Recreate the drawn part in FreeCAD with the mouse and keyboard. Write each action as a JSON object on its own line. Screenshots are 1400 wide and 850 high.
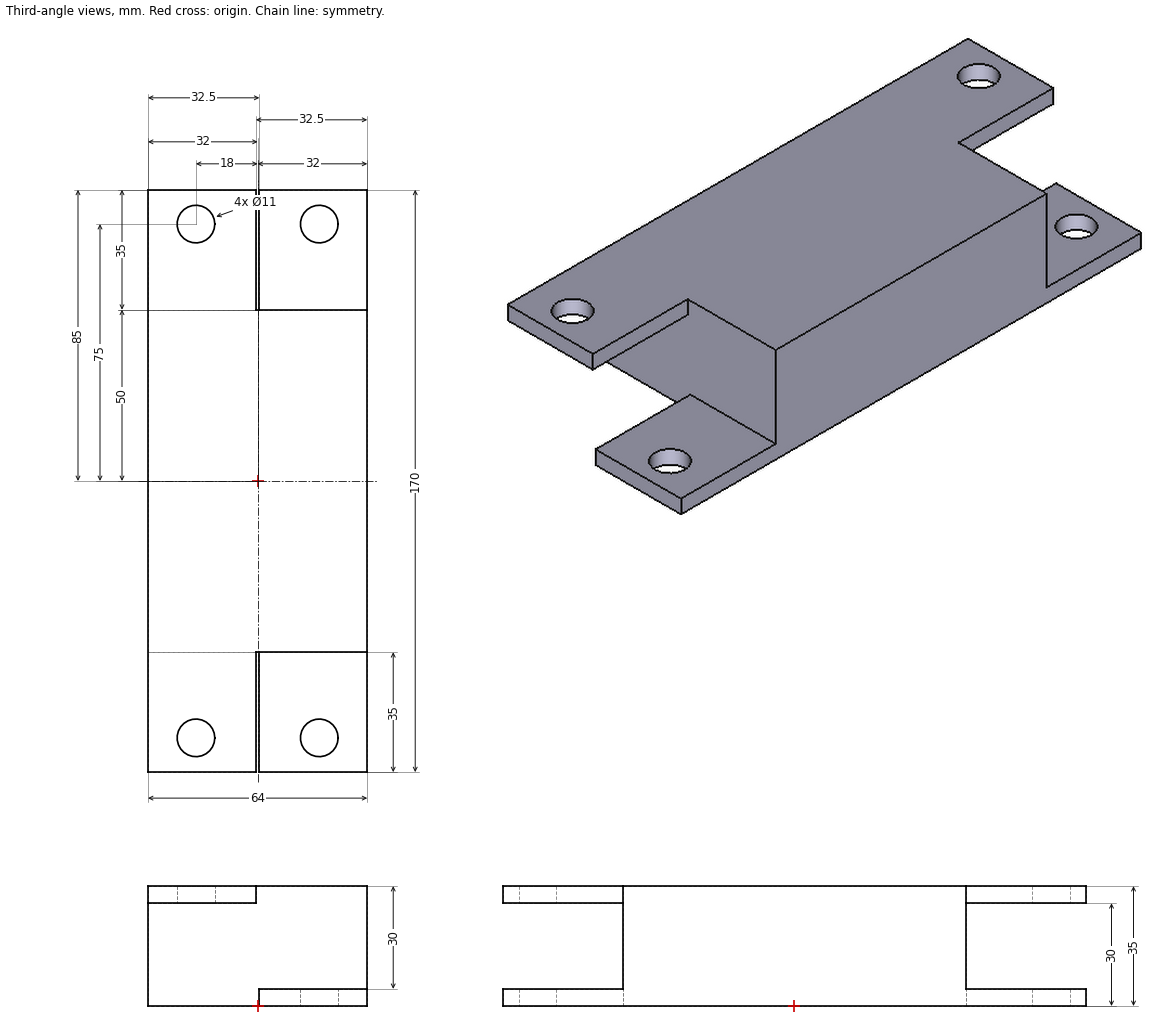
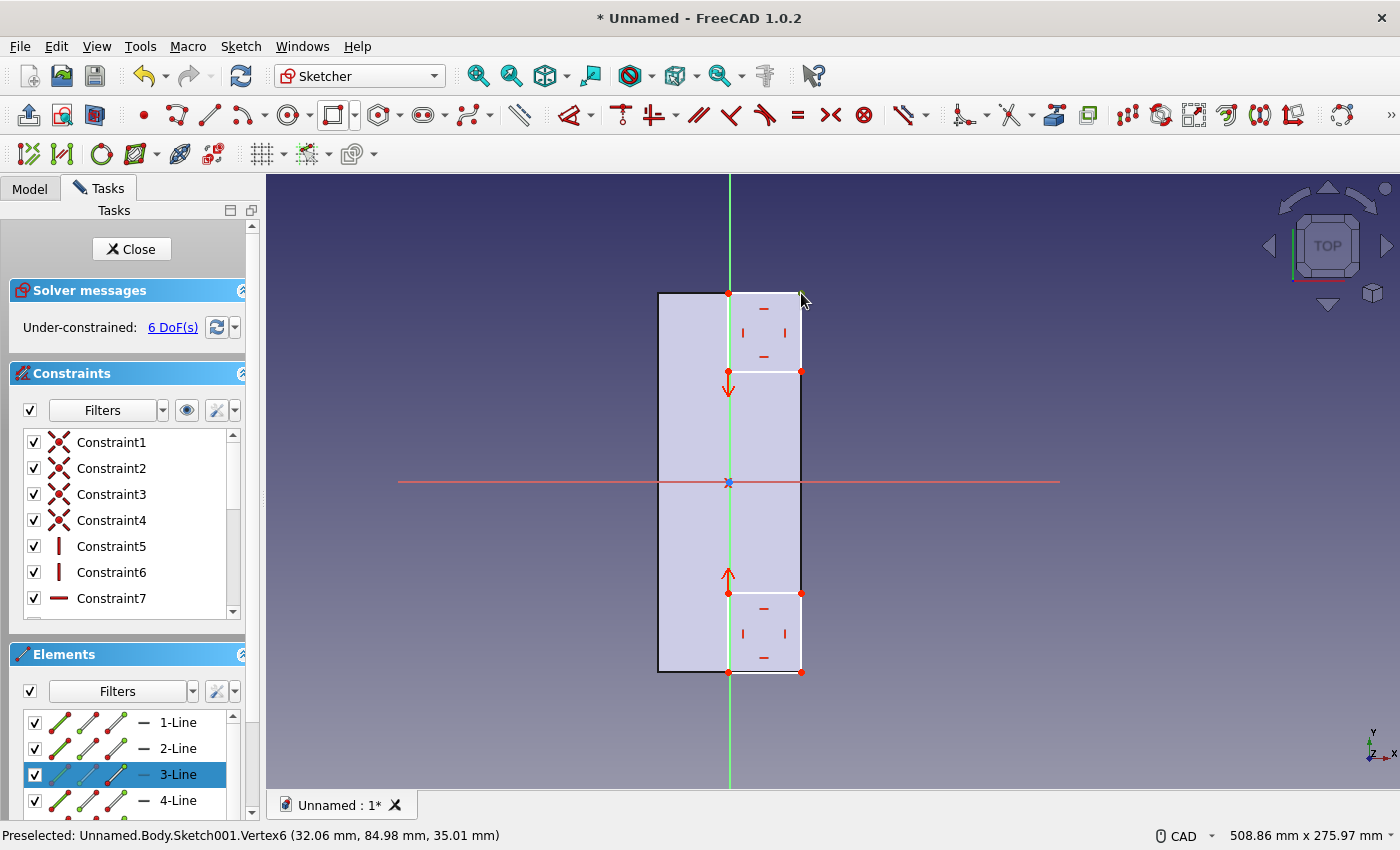
{"action": "left_click", "coordinate": [801, 673]}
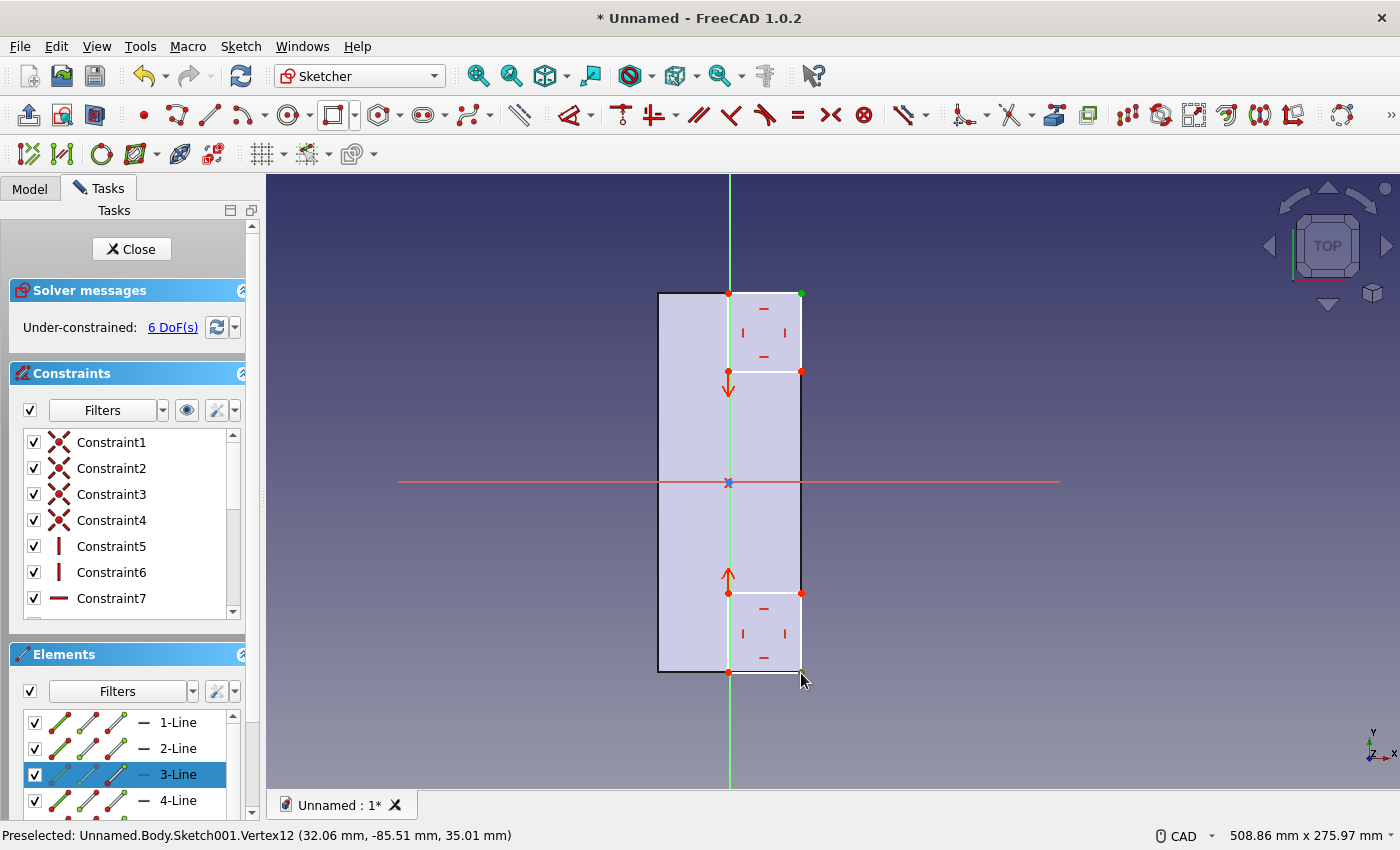
{"action": "left_click", "coordinate": [428, 482]}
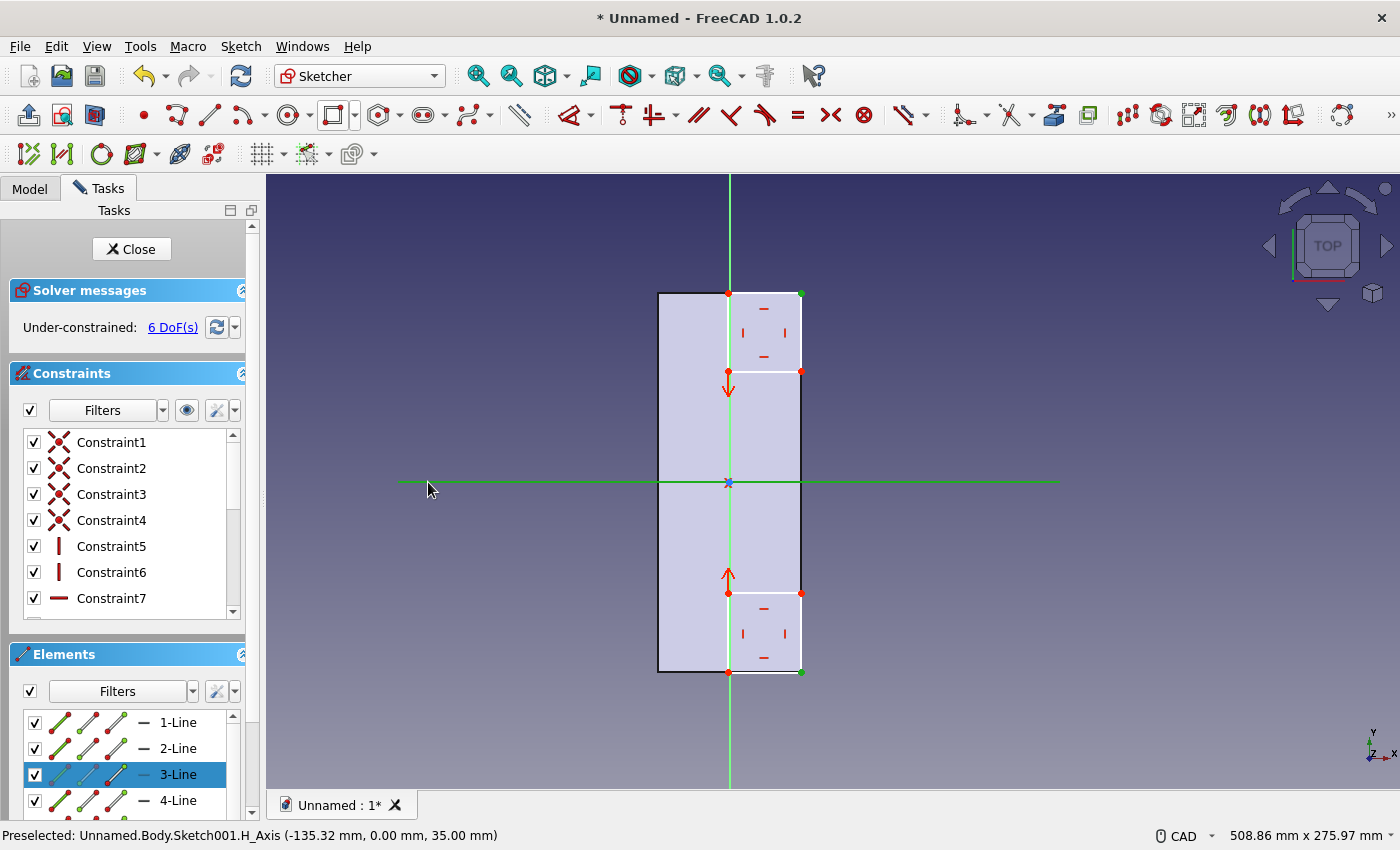
{"action": "left_click", "coordinate": [831, 116]}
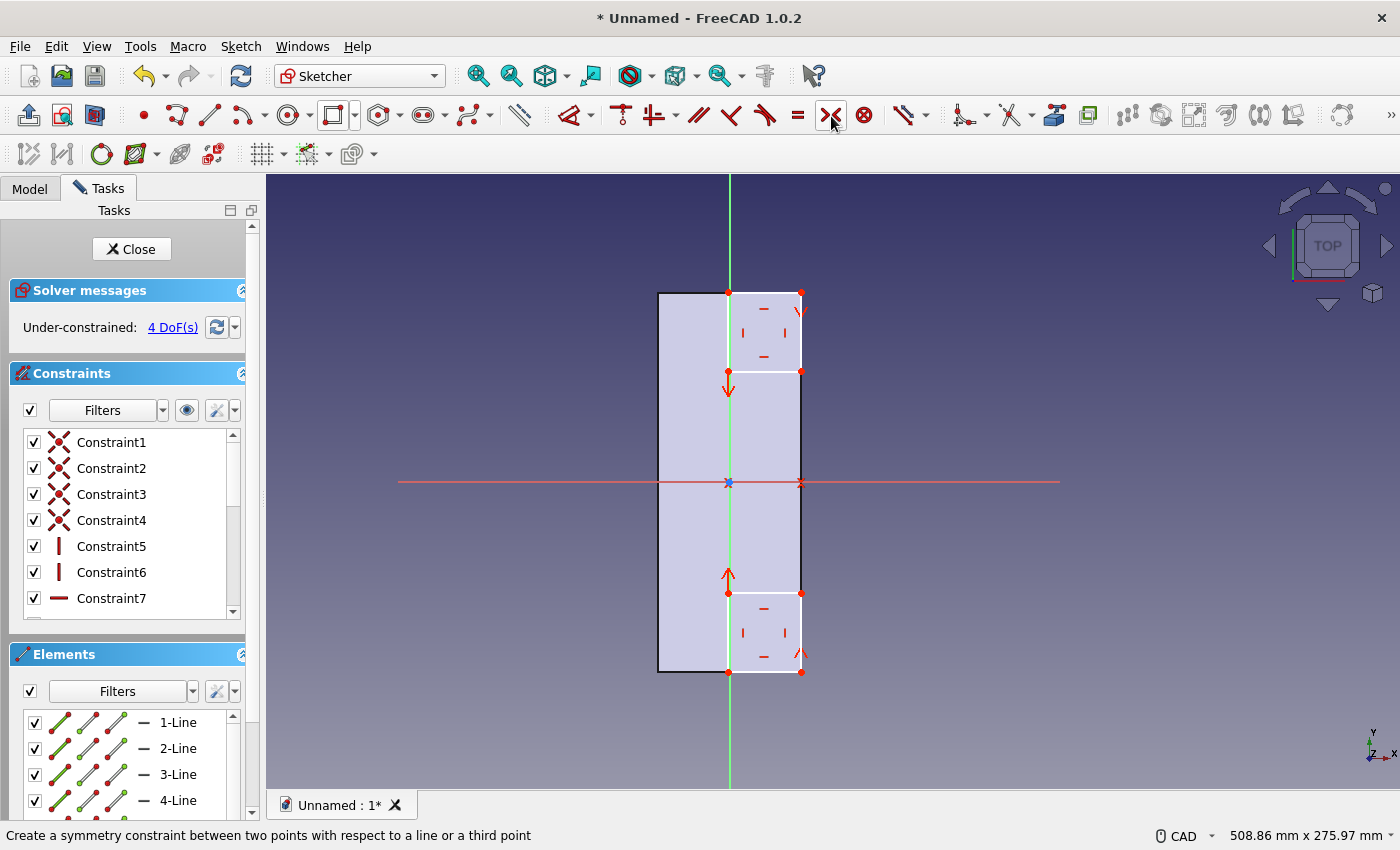
{"action": "left_click", "coordinate": [728, 316]}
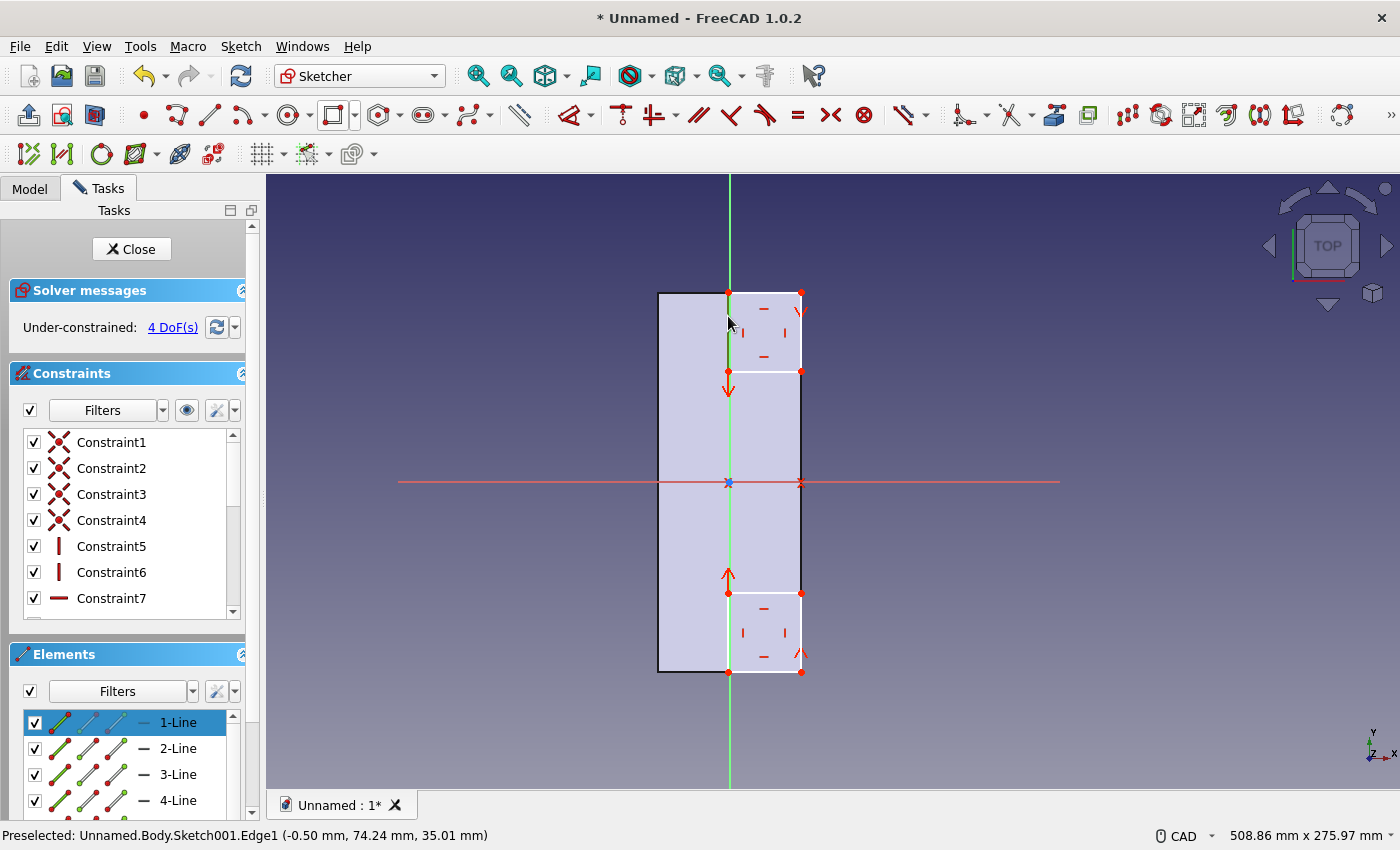
{"action": "key", "text": "i"}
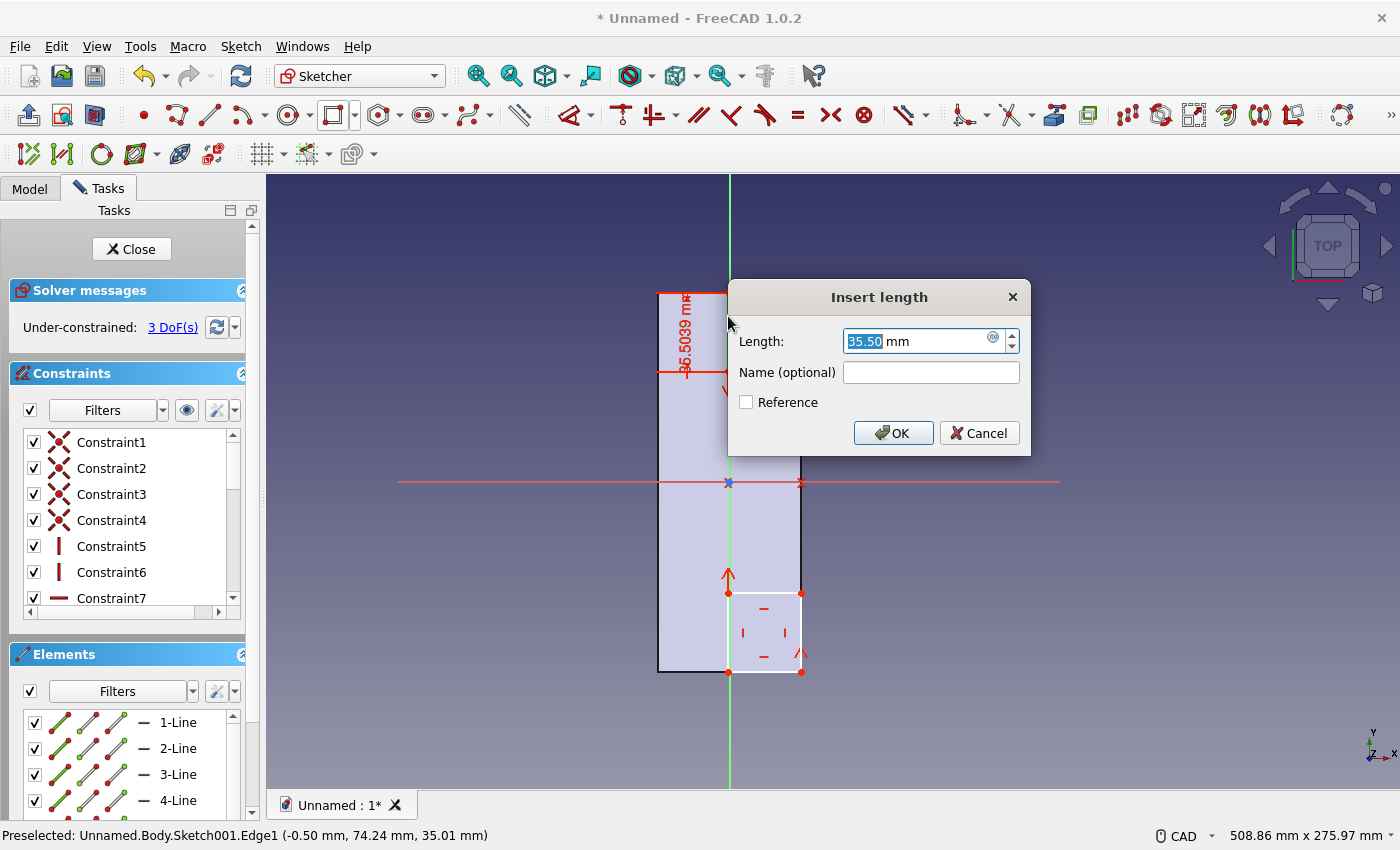
{"action": "type", "text": "35"}
{"action": "key", "text": "Return"}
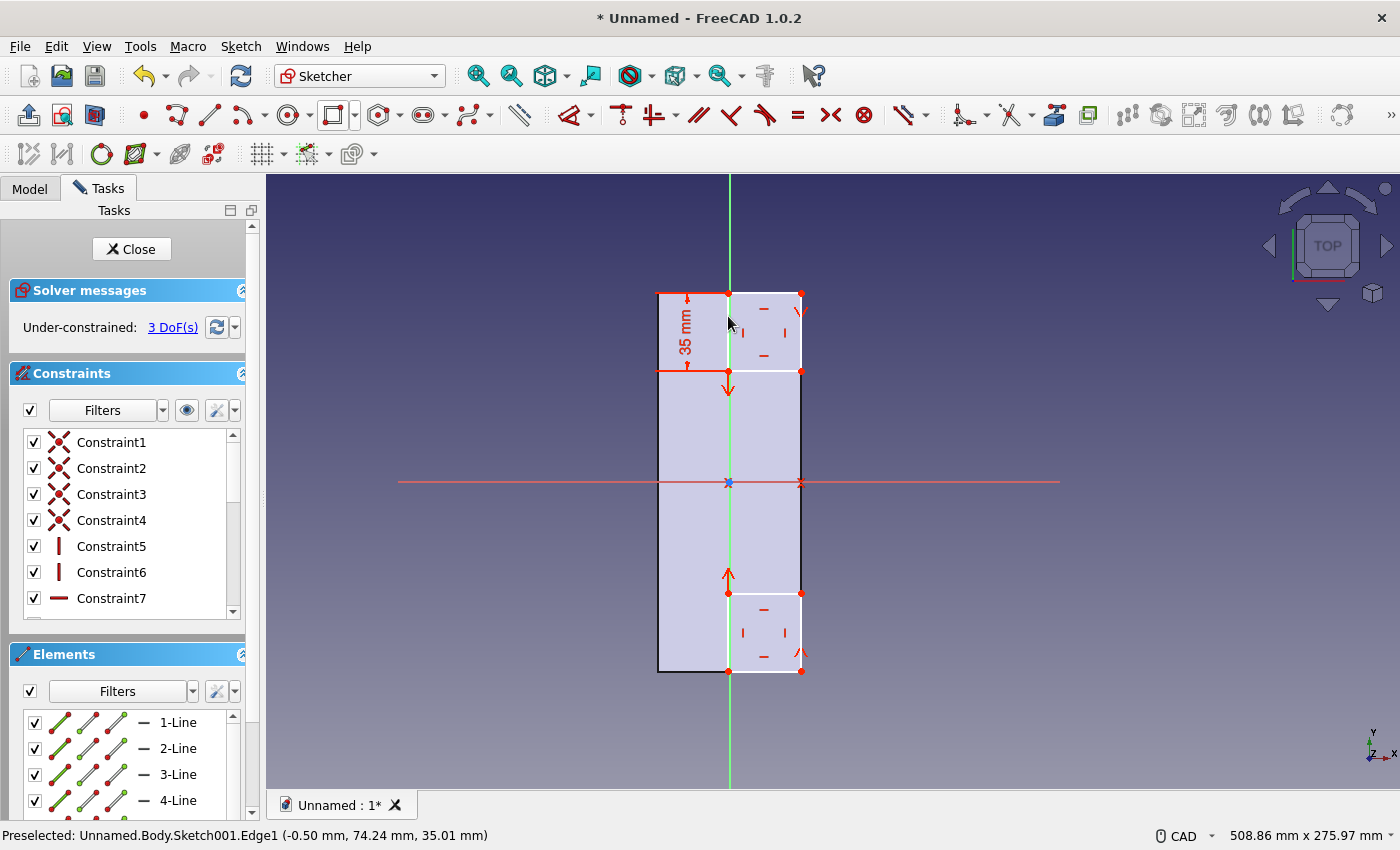
{"action": "left_click", "coordinate": [728, 293]}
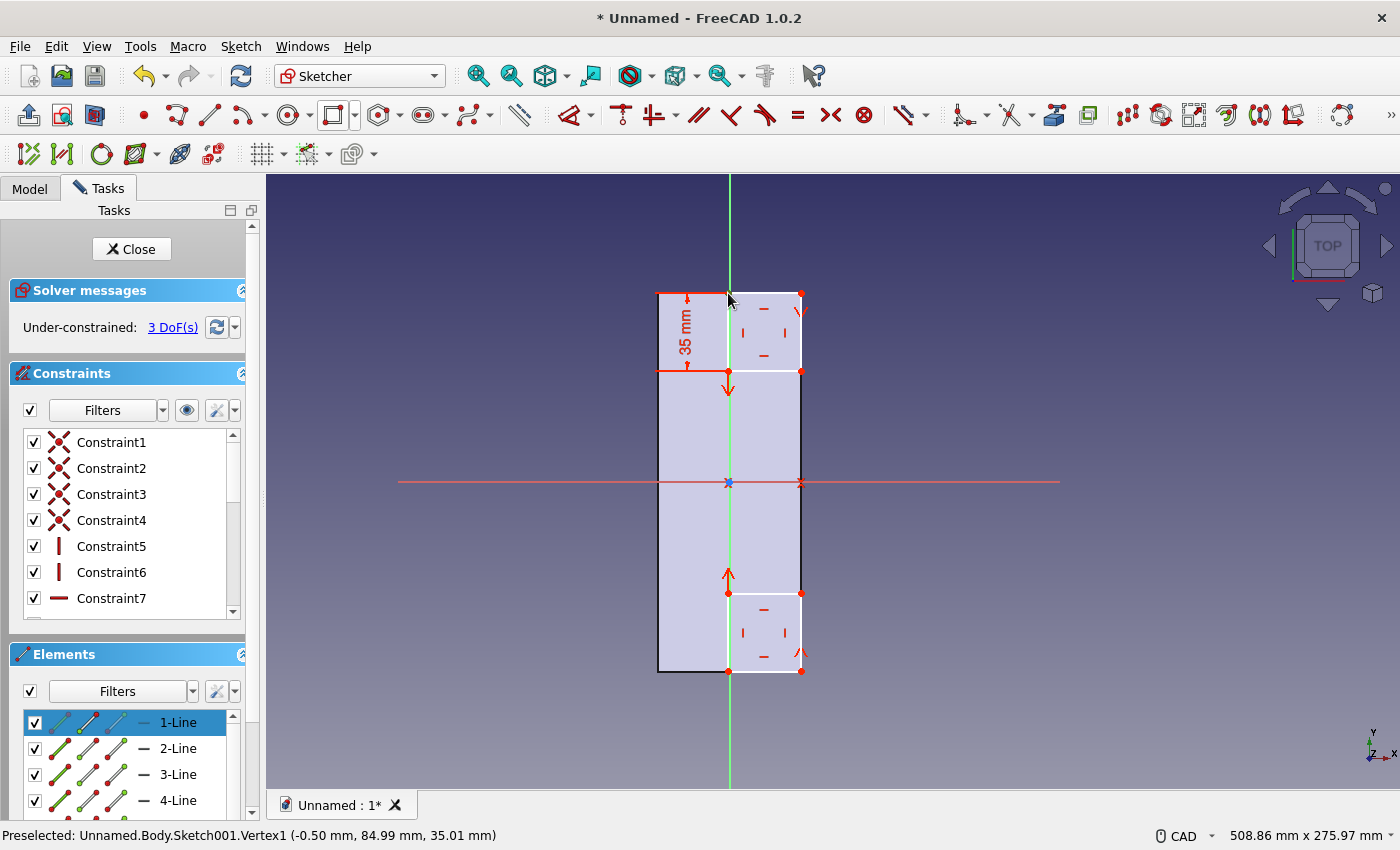
{"action": "left_click", "coordinate": [590, 116]}